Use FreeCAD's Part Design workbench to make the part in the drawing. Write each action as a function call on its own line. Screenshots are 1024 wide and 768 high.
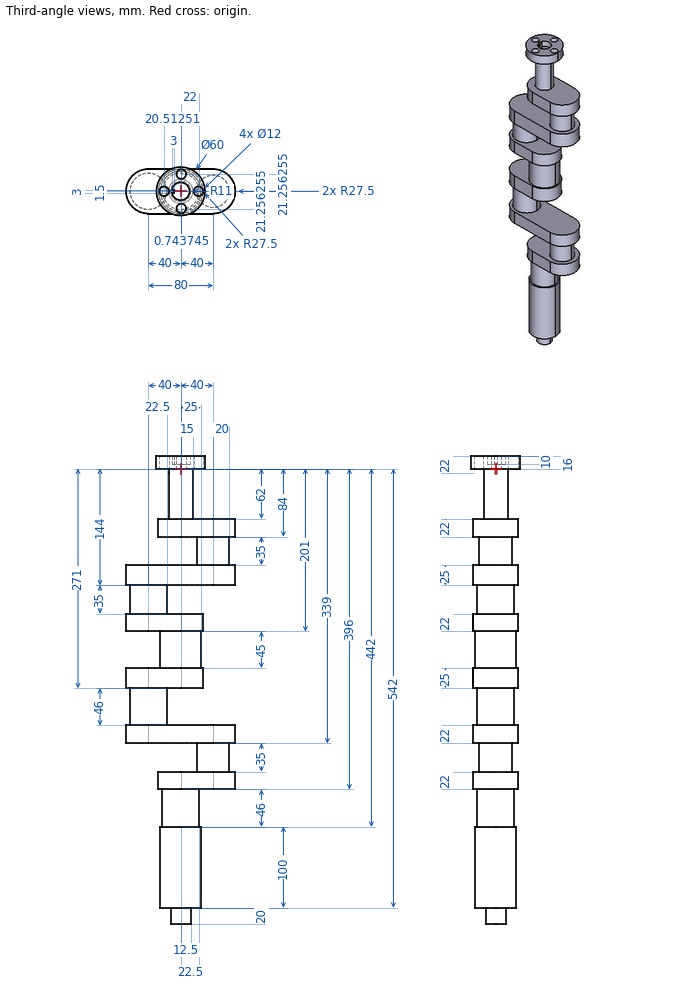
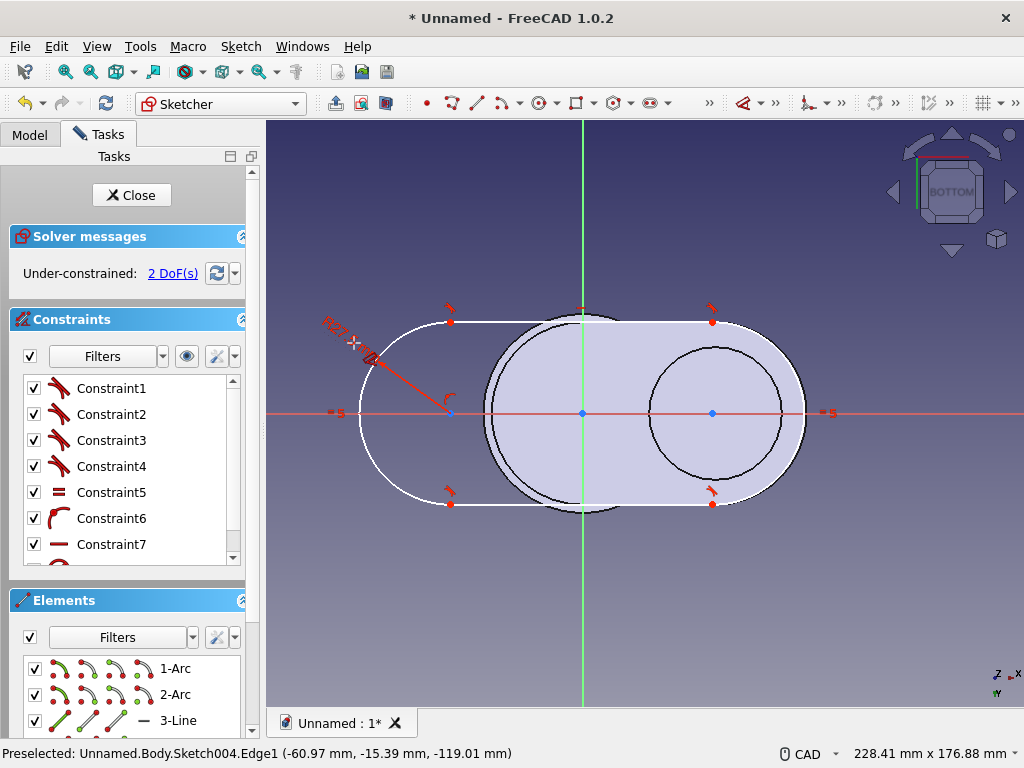
click(529, 322)
click(522, 288)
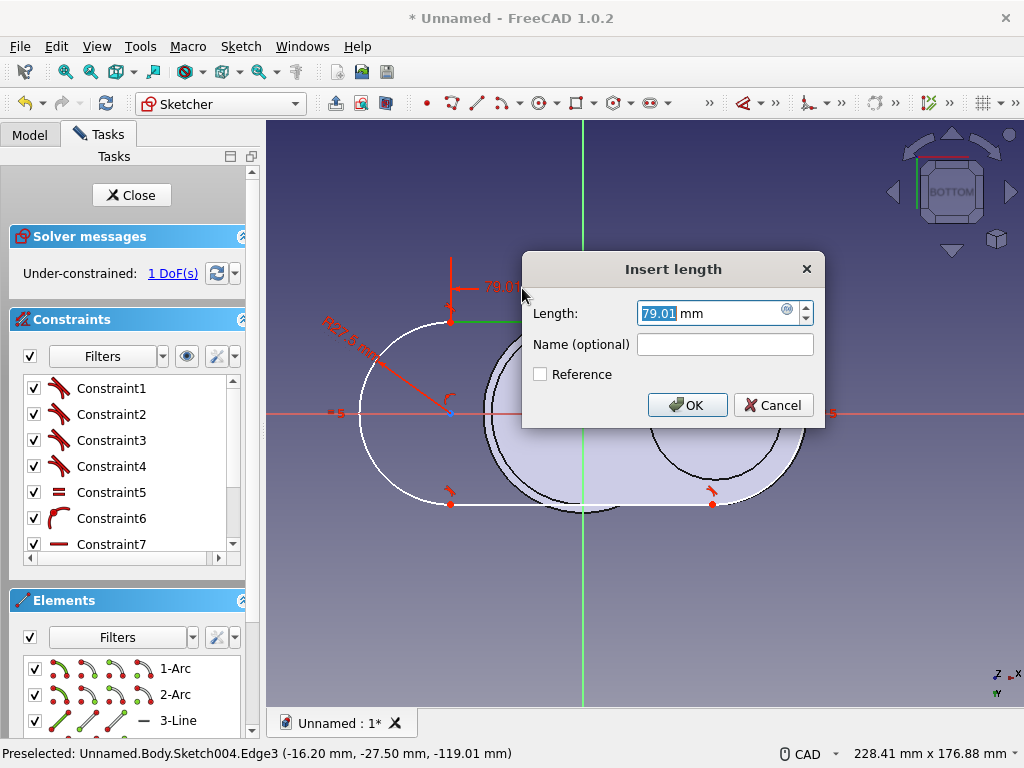
text(80)
key(Return)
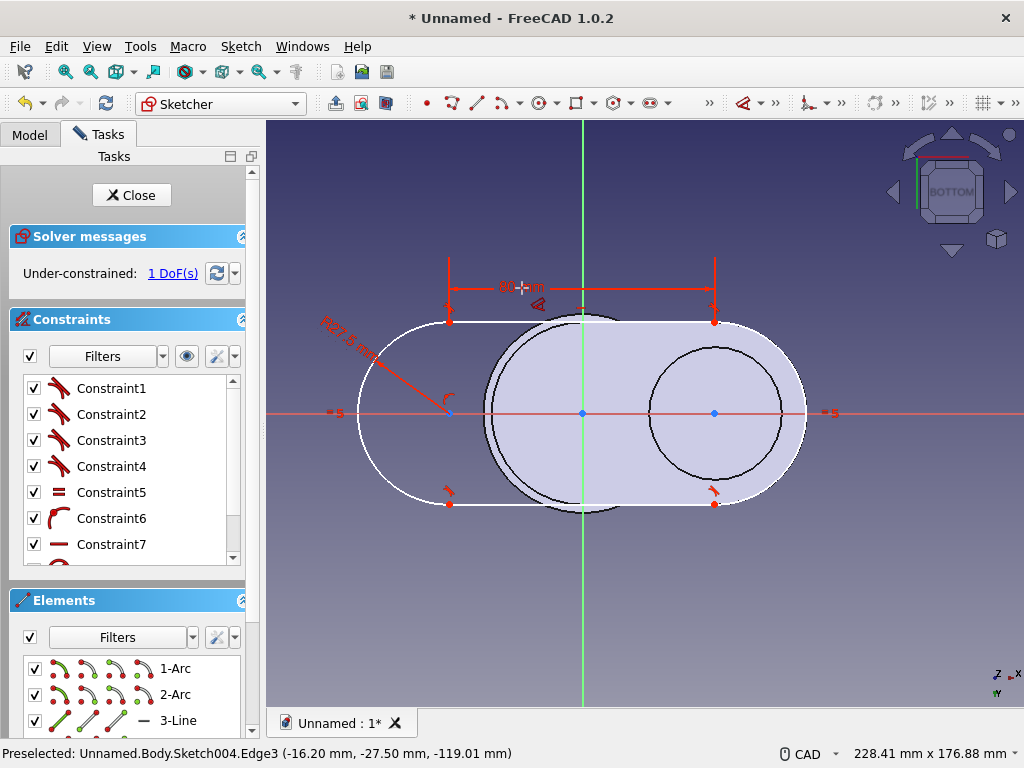
click(449, 322)
click(516, 447)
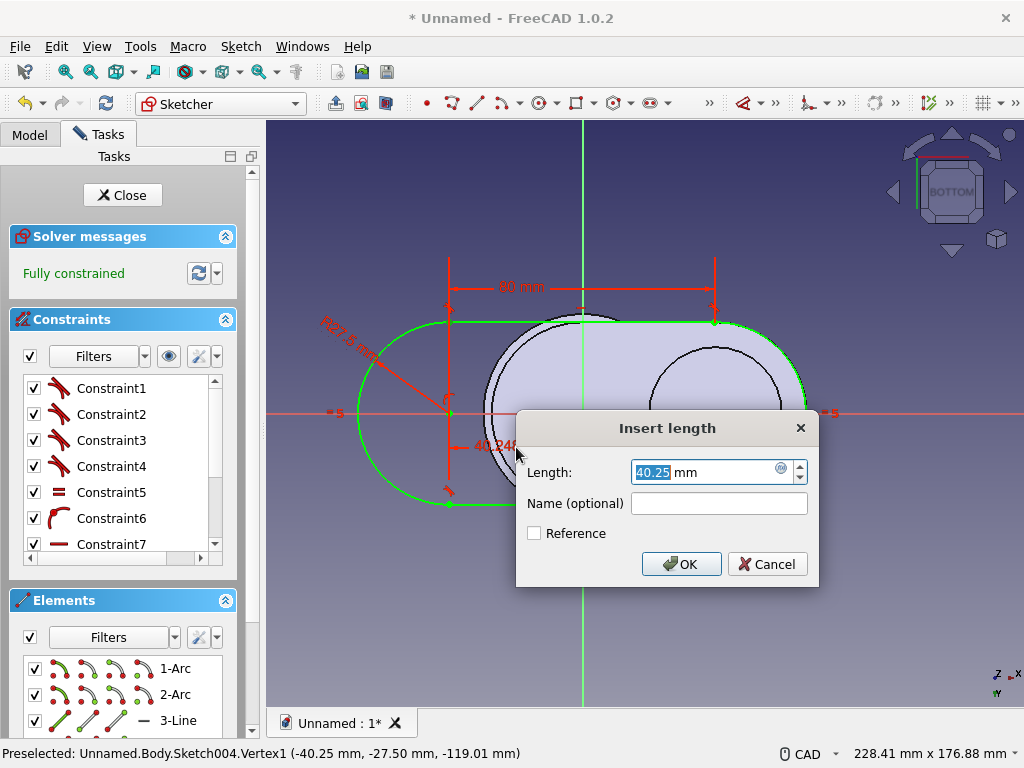
text(40)
key(Return)
key(Escape)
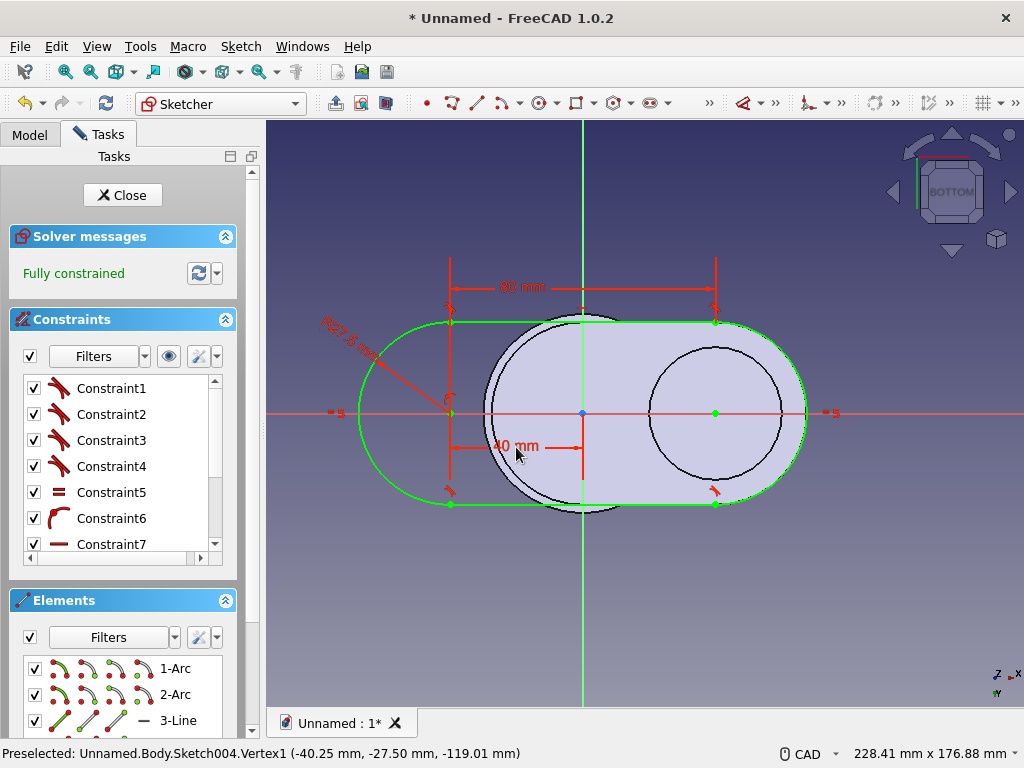
click(123, 195)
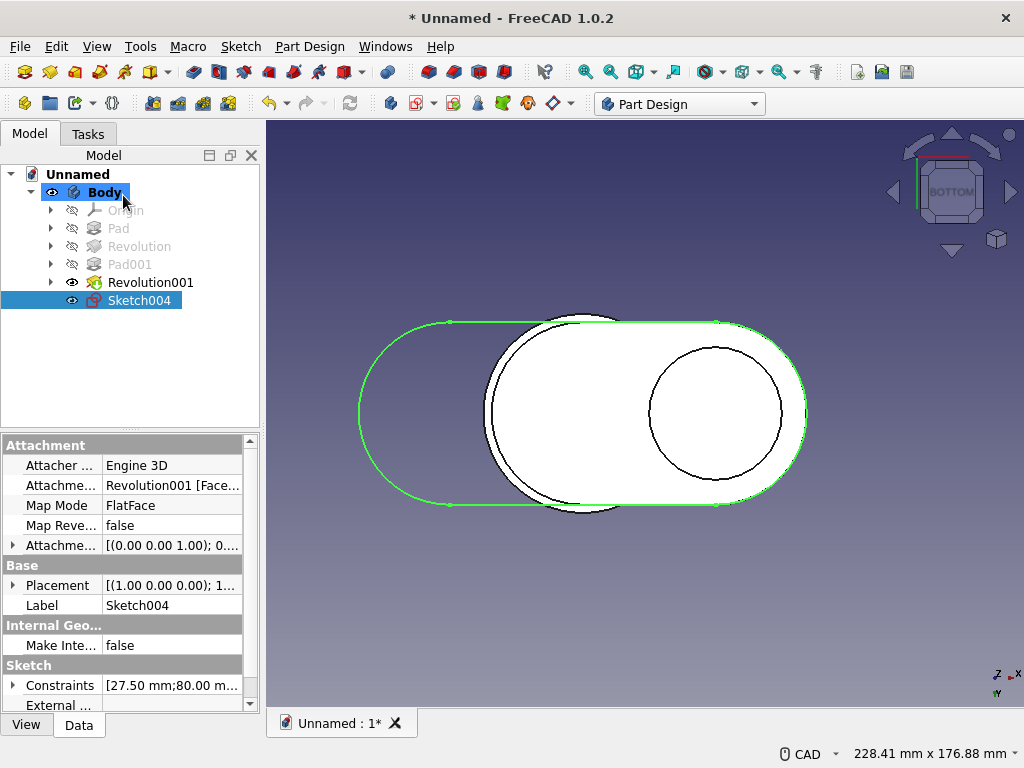
click(25, 72)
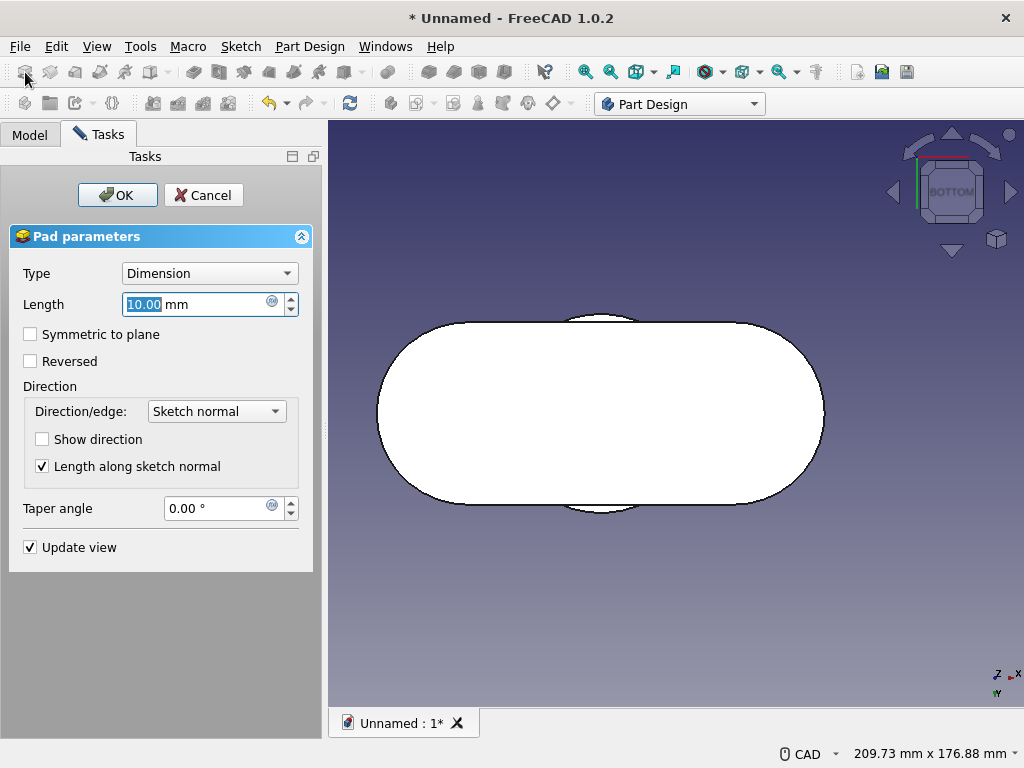
text(25)
key(Tab)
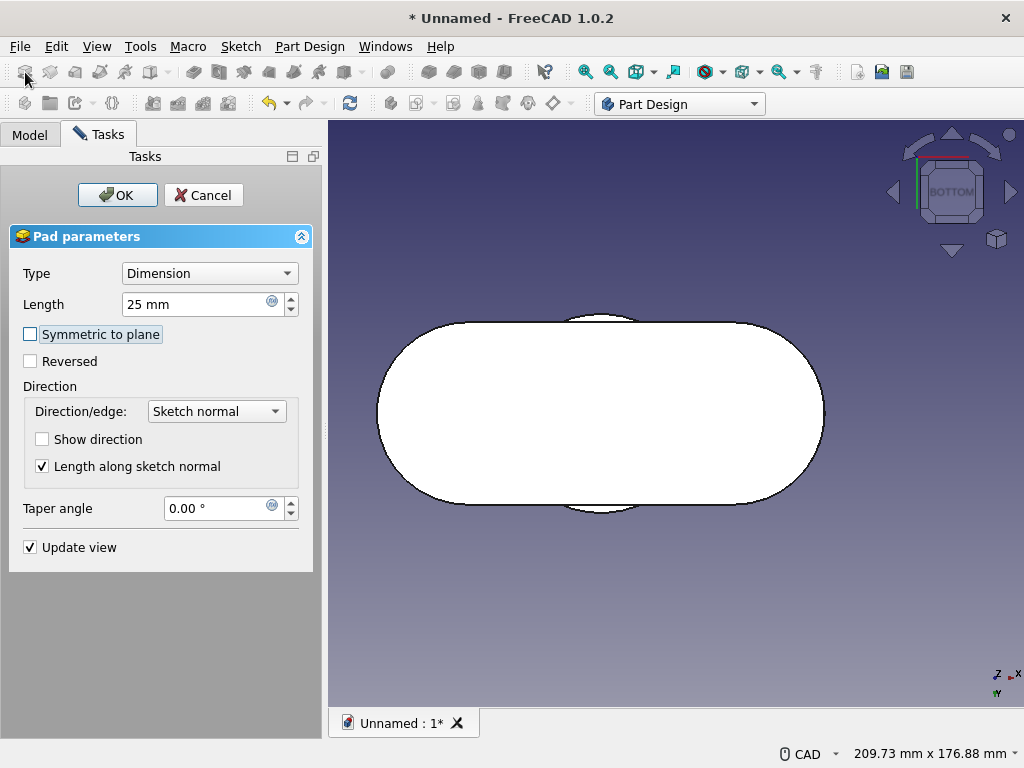
click(118, 195)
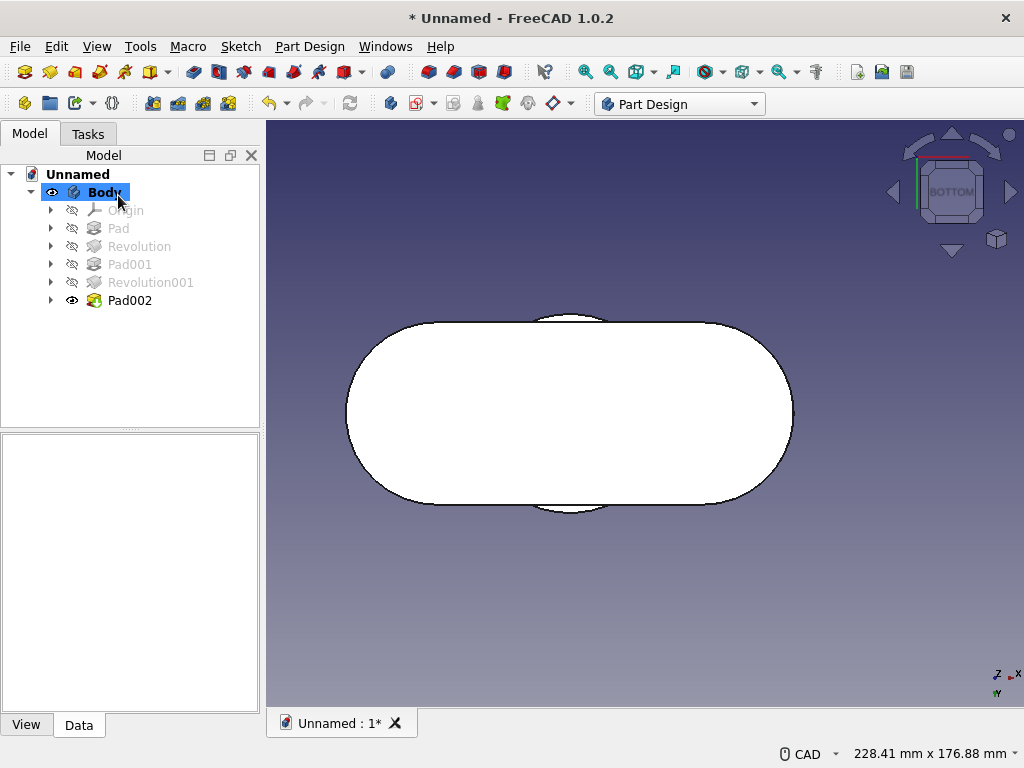
click(416, 104)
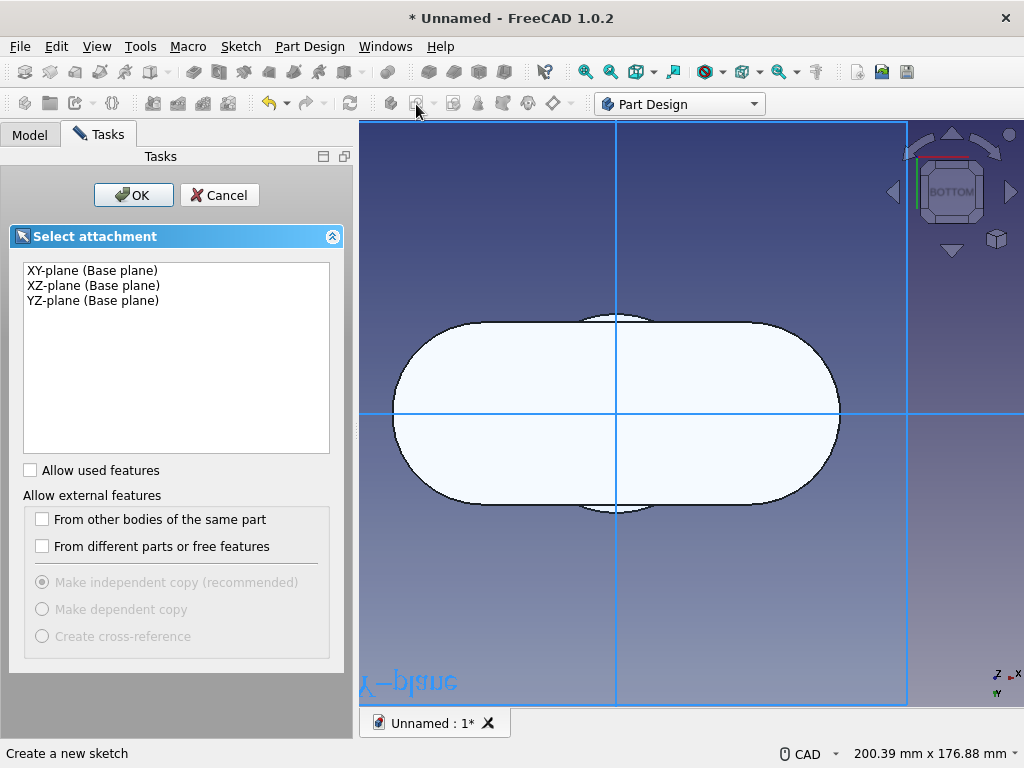
click(84, 286)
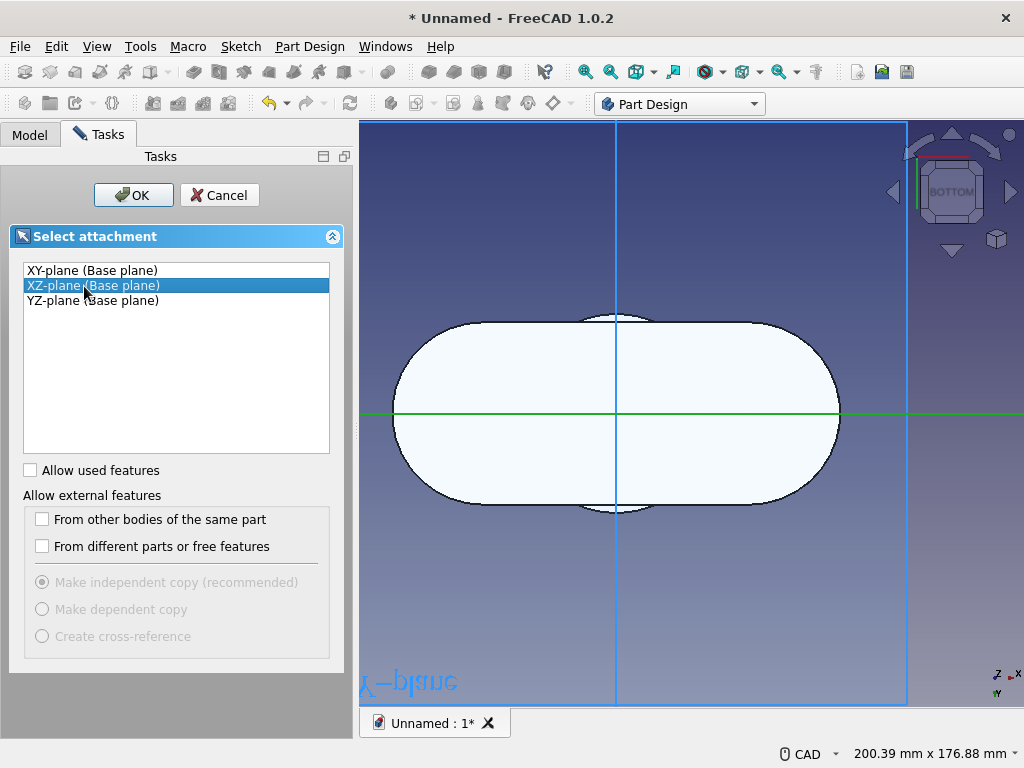
click(134, 195)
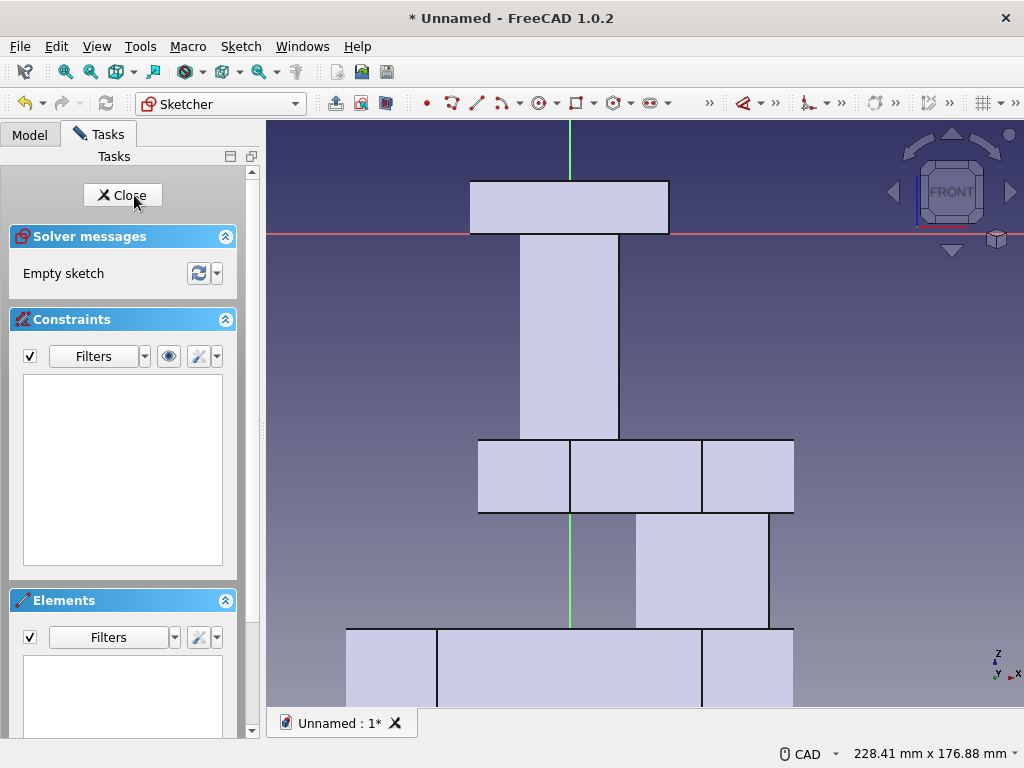
key(q)
key(s)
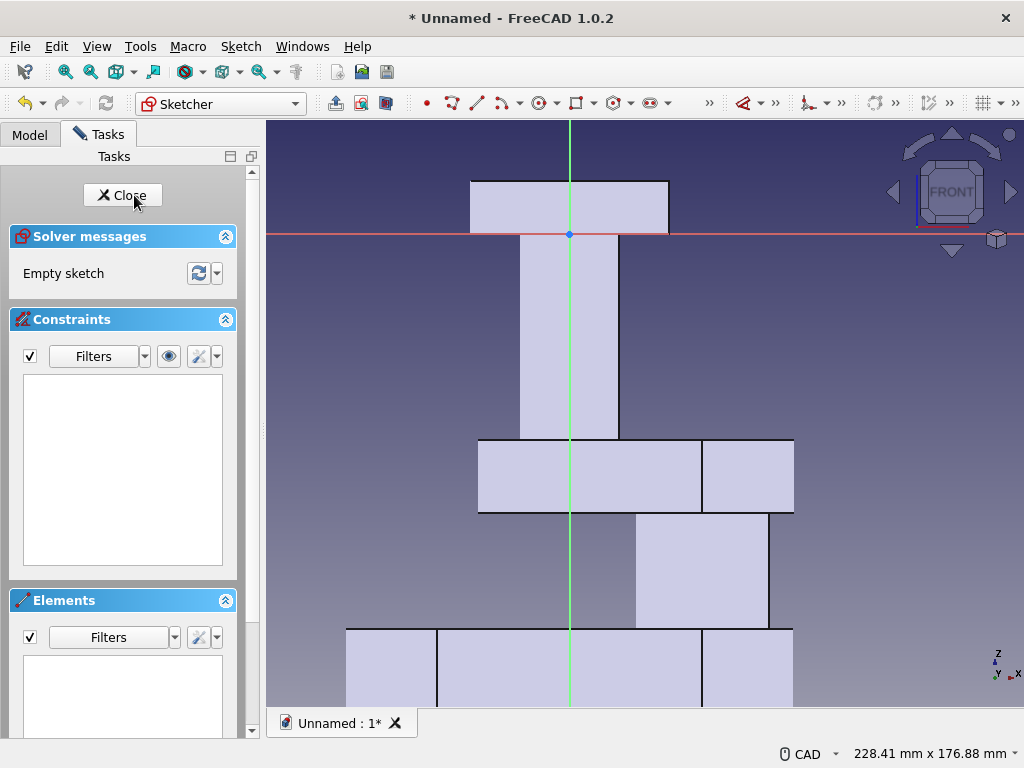
scroll(576, 414, down, 5)